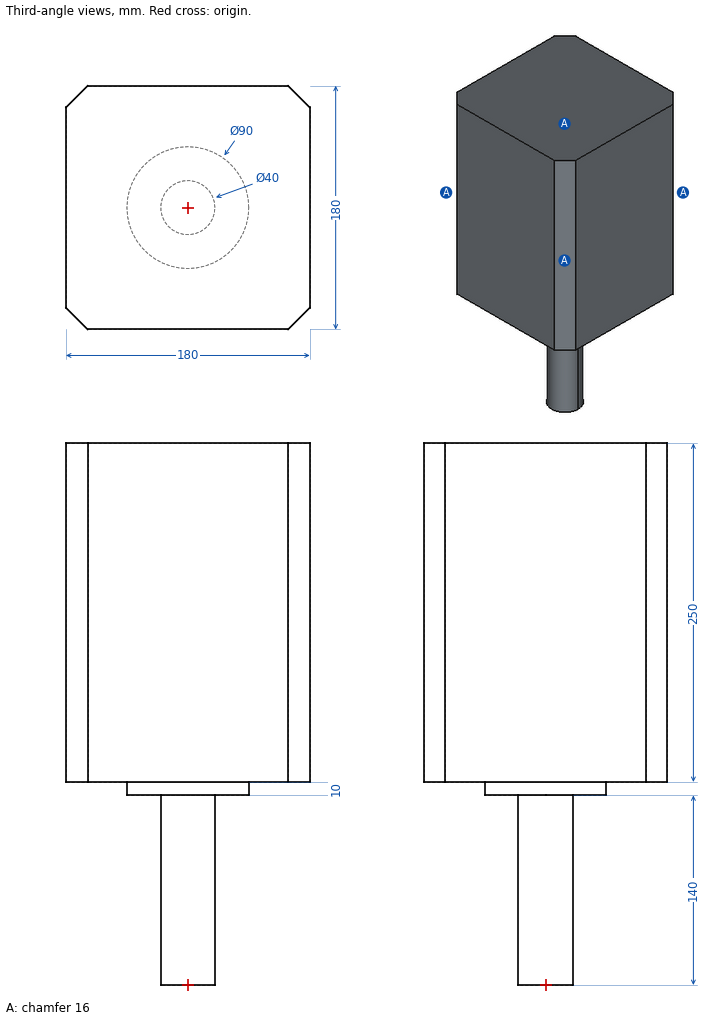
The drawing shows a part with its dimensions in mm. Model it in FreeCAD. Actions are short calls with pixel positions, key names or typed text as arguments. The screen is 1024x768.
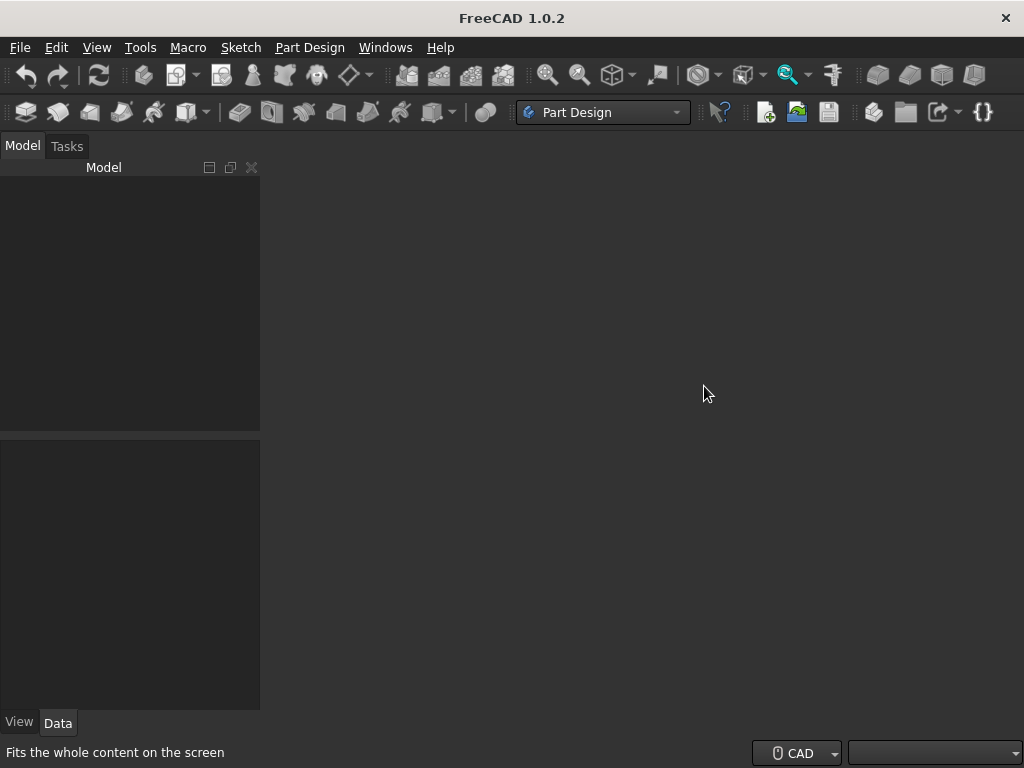
click(766, 112)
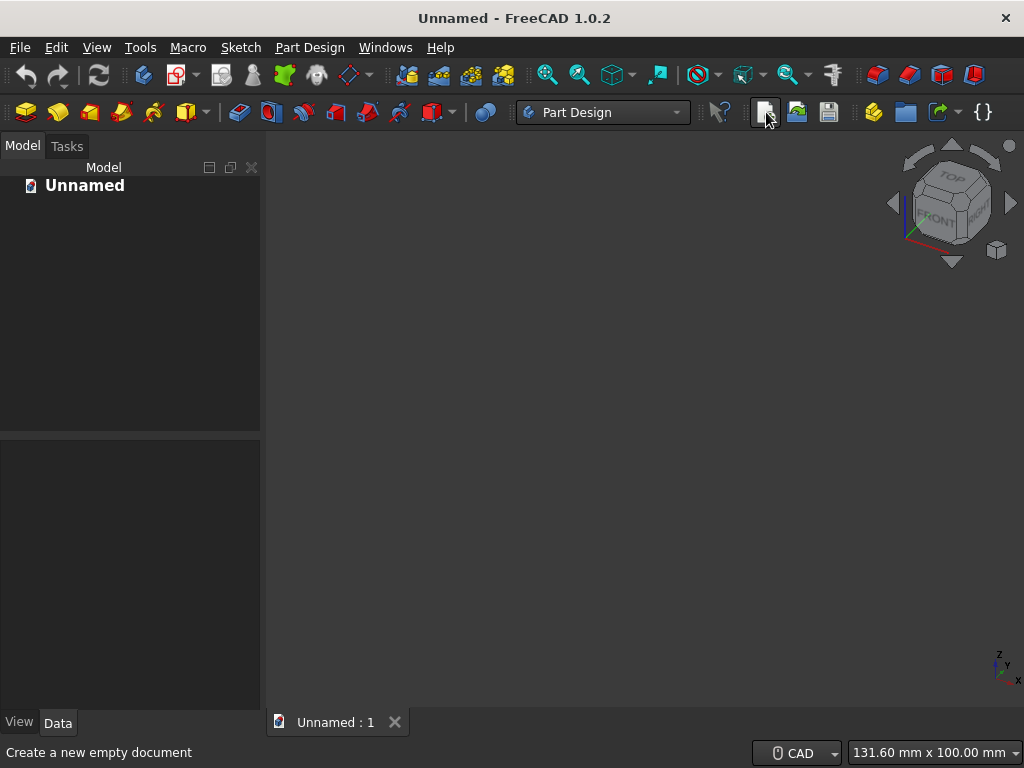
click(176, 76)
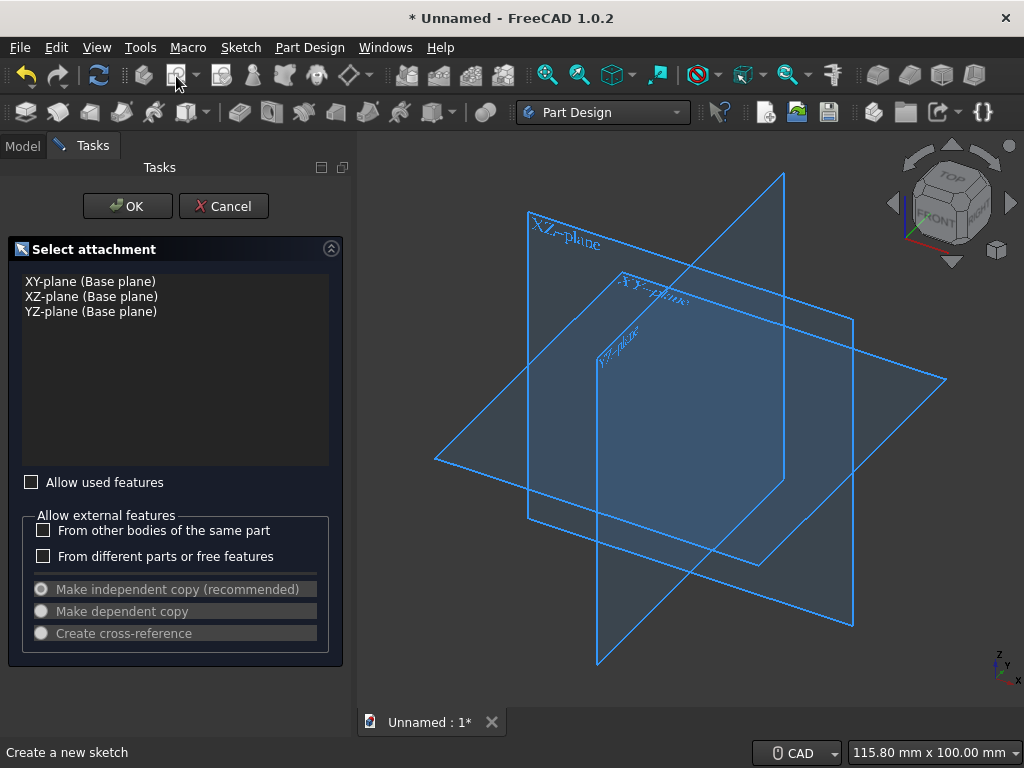
click(82, 282)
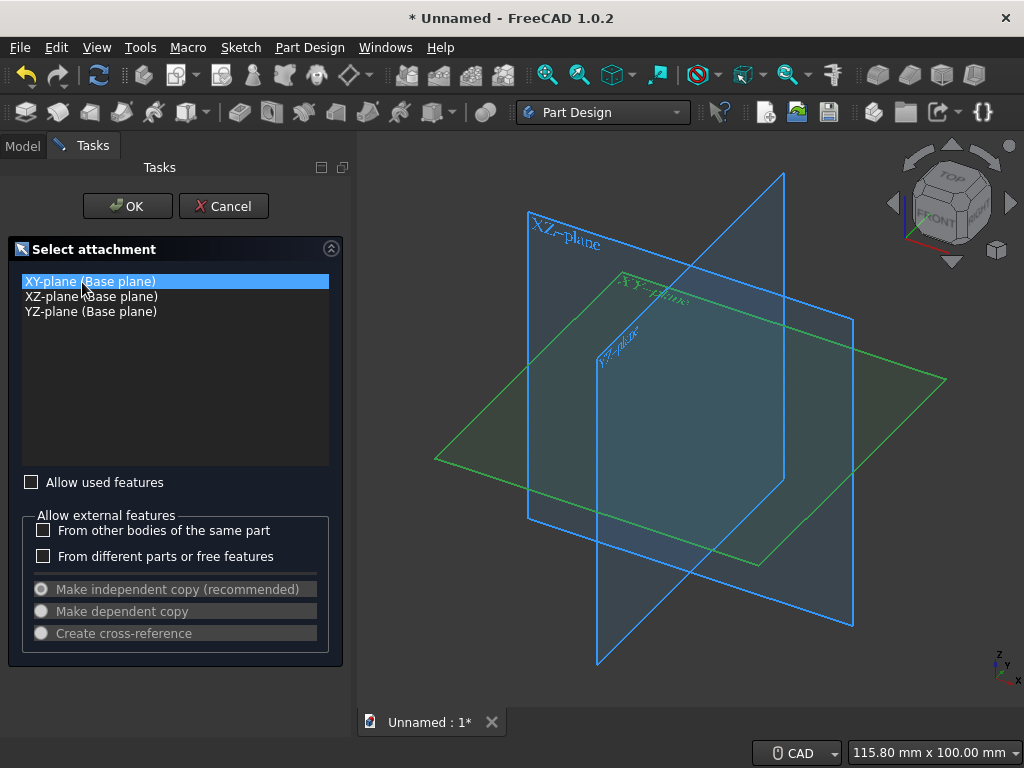
click(128, 206)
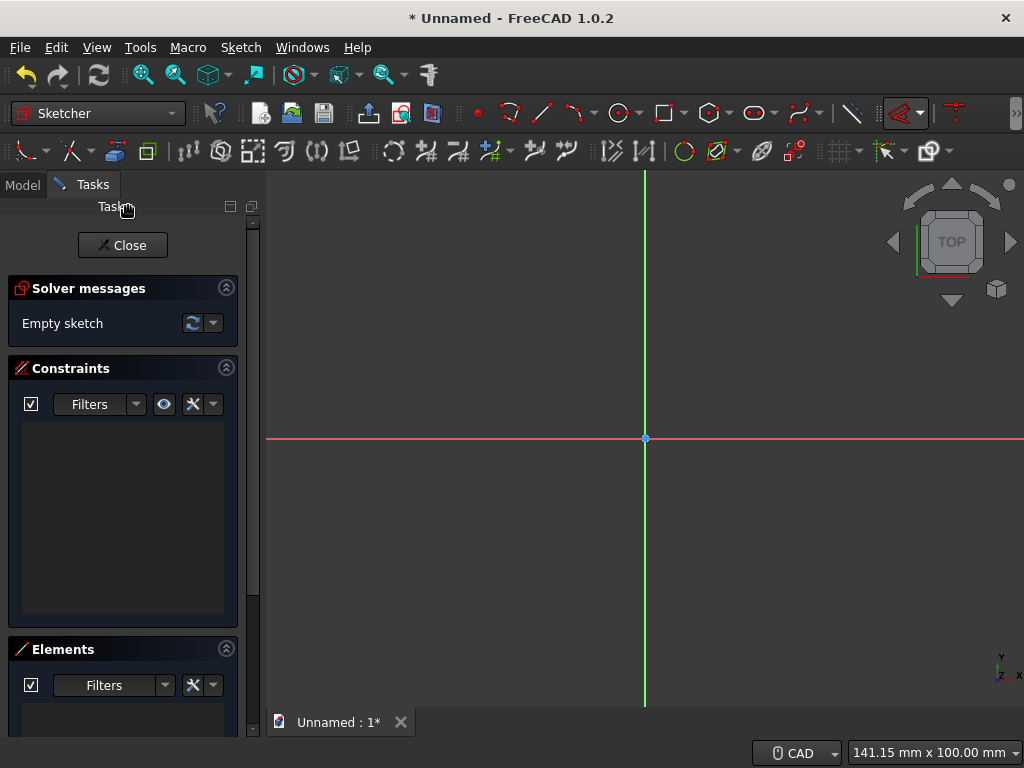
scroll(784, 439, up, 2)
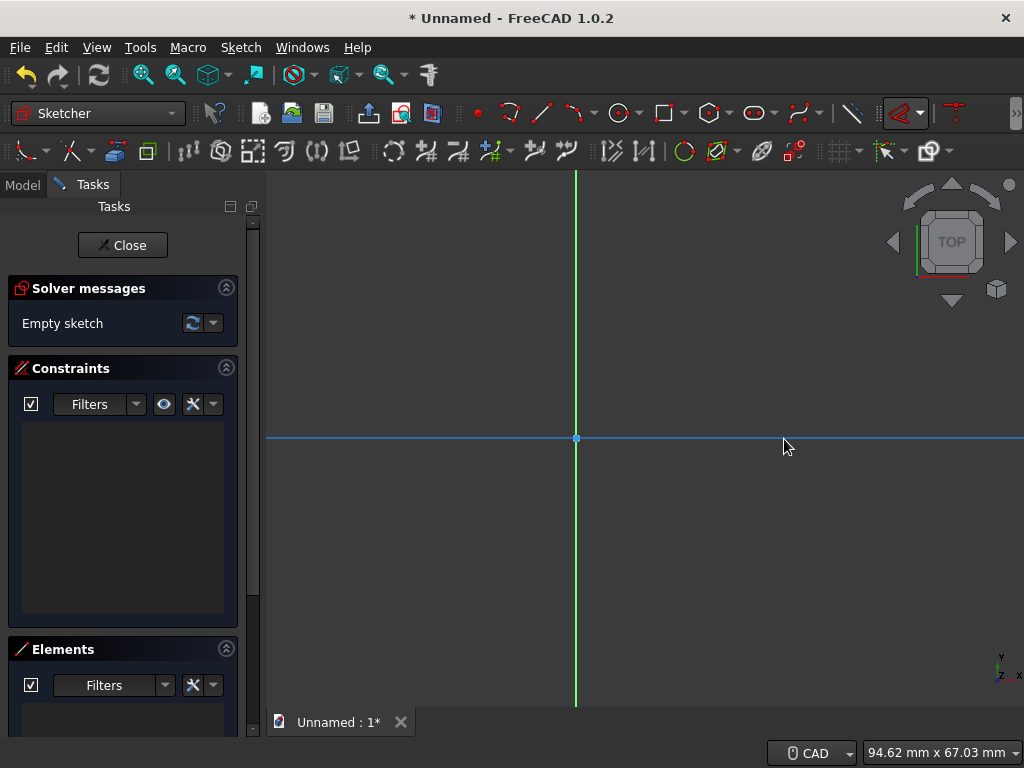
click(620, 114)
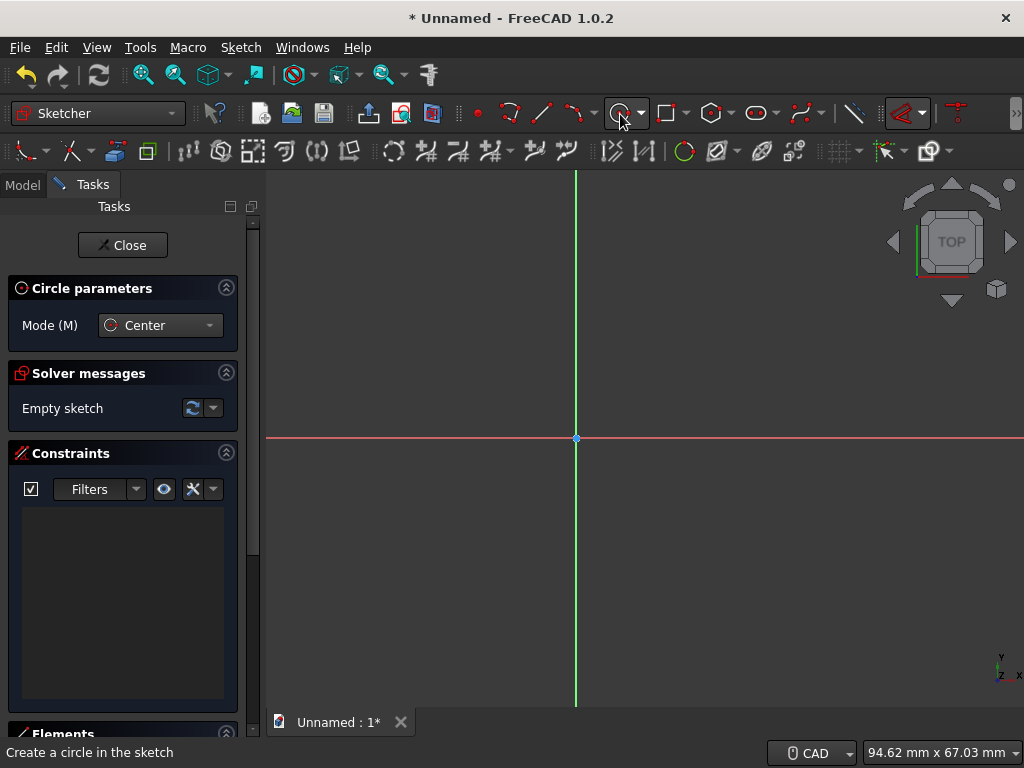
click(576, 438)
click(690, 325)
key(Escape)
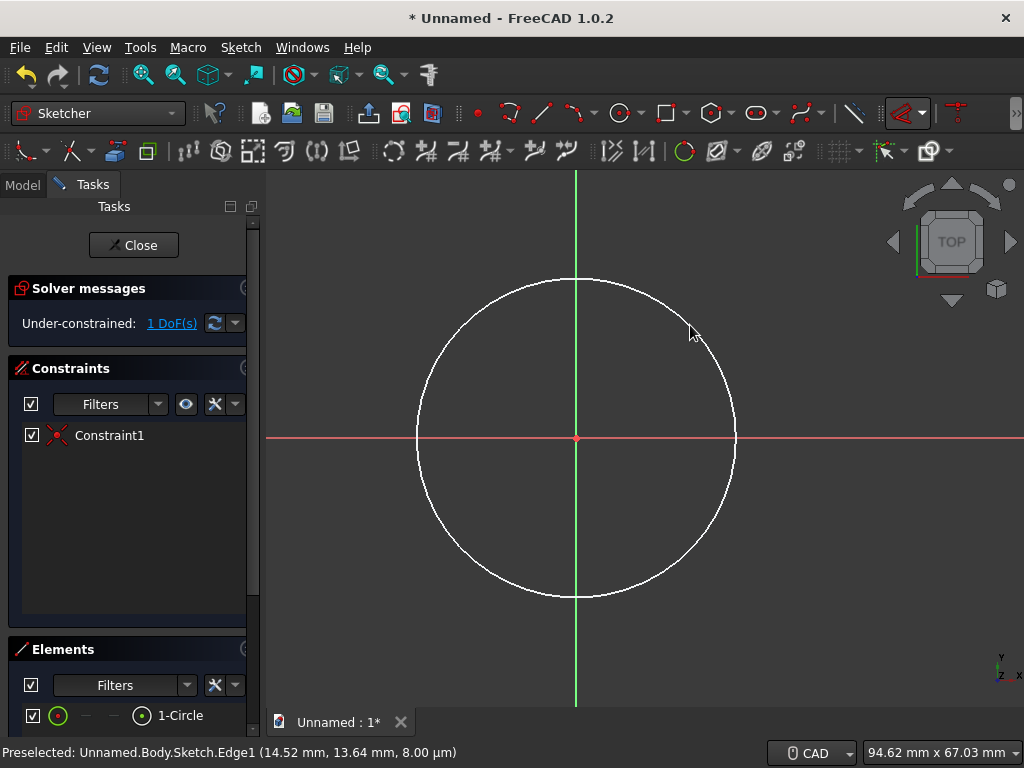
click(902, 114)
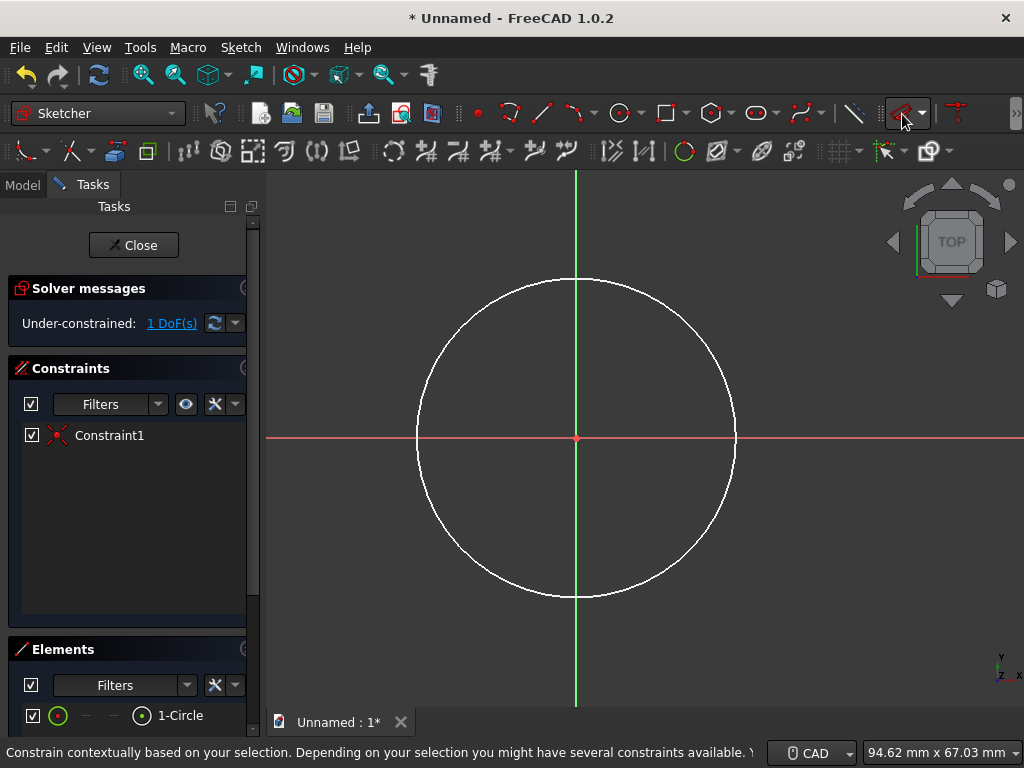
click(689, 325)
click(712, 302)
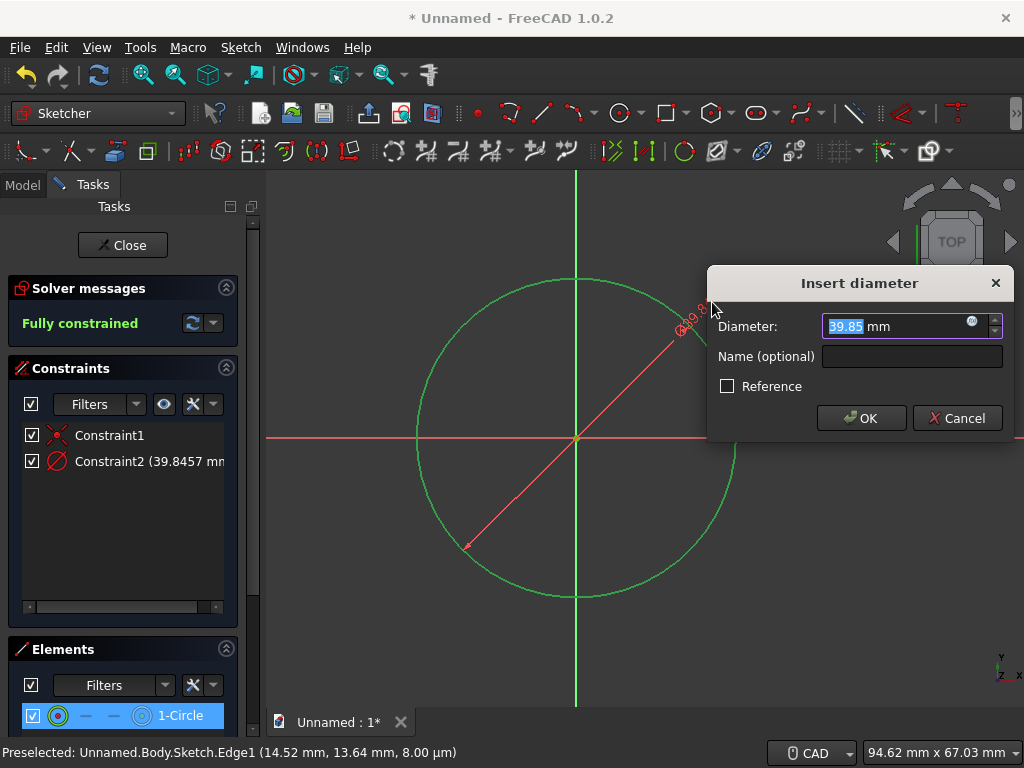
text(40)
key(Return)
key(Escape)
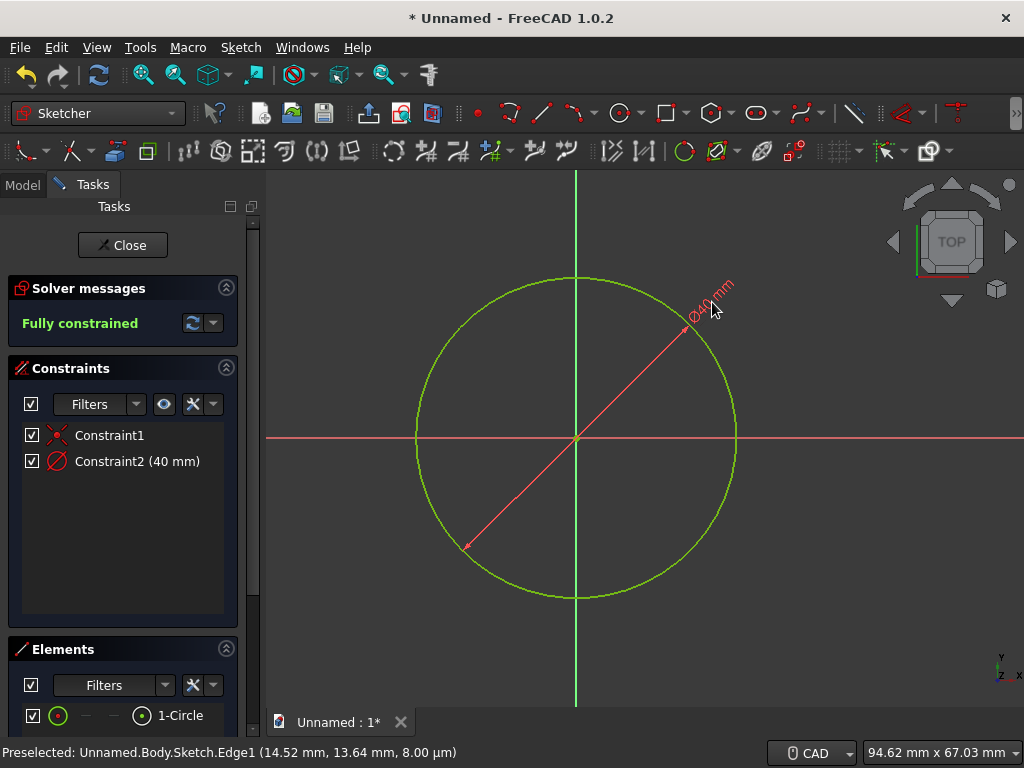
click(123, 245)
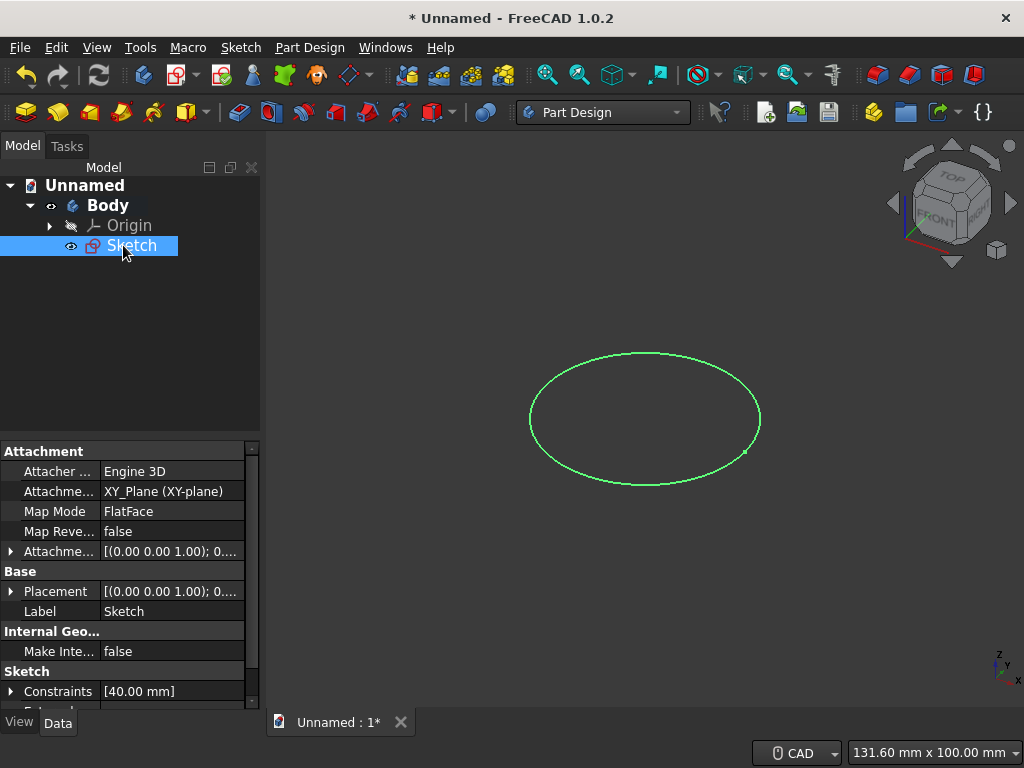
click(26, 112)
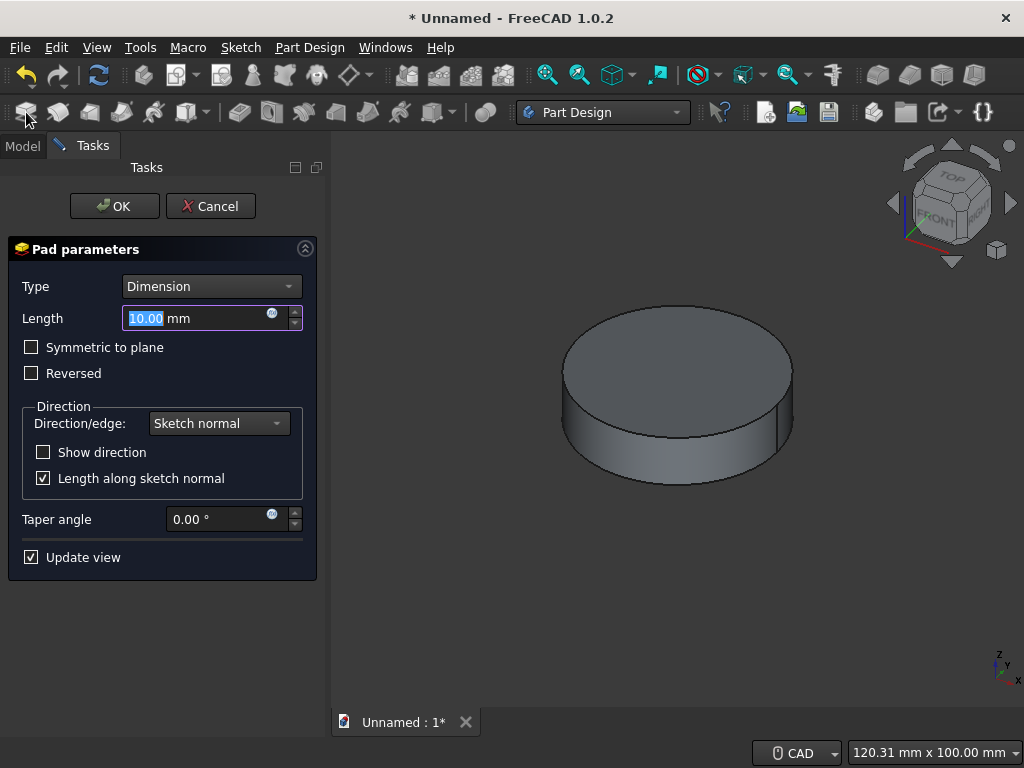
text(140)
key(Tab)